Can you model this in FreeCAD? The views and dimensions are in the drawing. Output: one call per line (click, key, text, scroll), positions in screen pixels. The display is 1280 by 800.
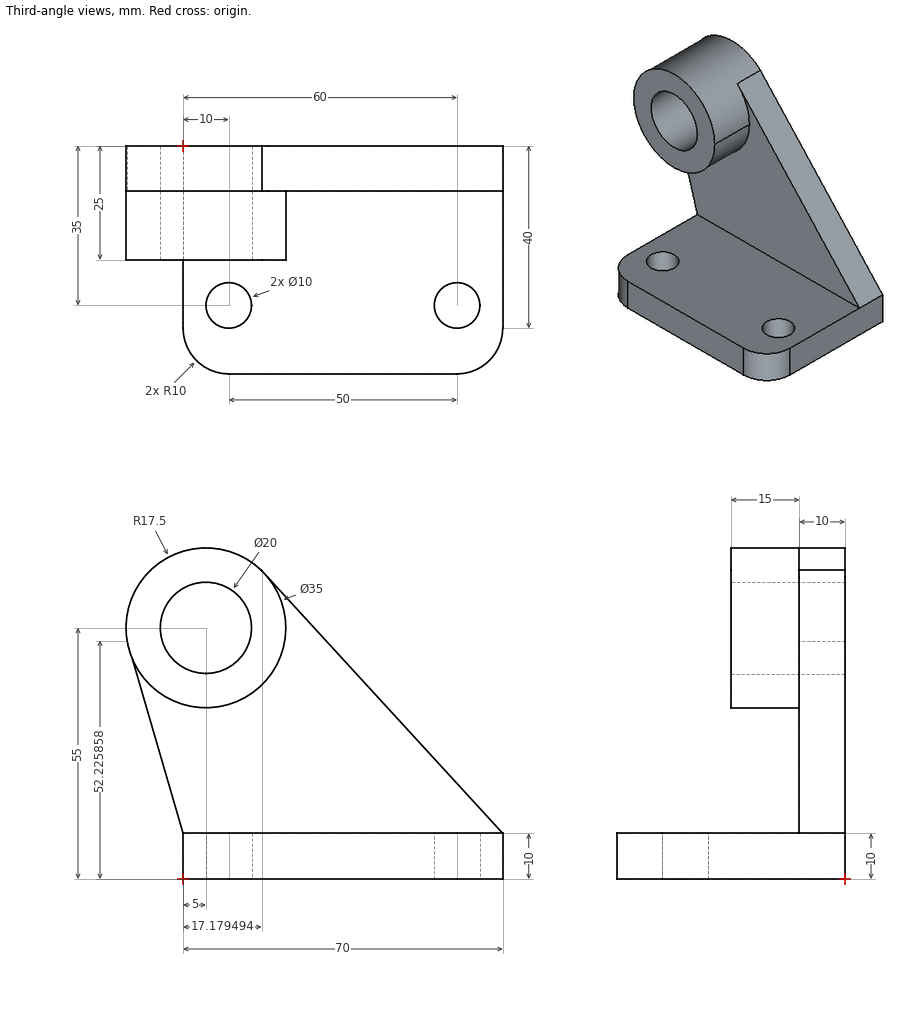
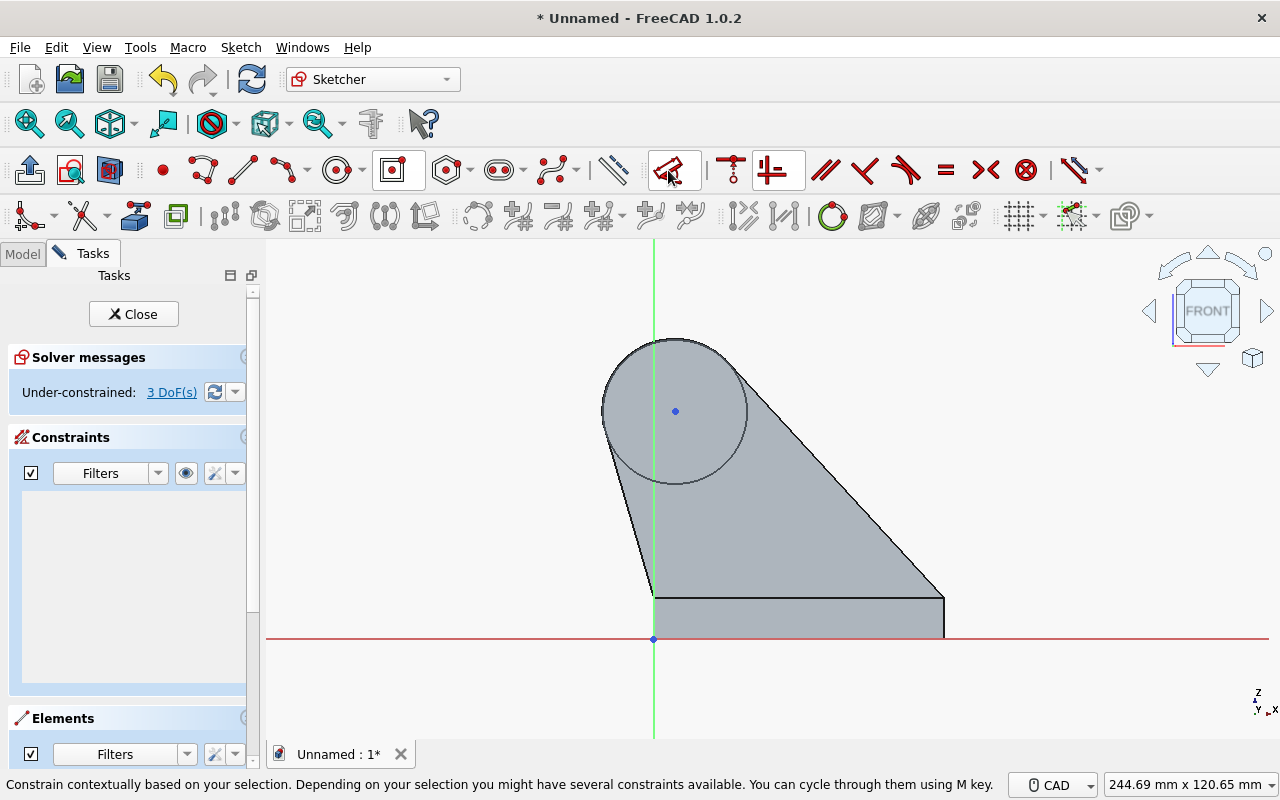
click(726, 361)
click(749, 338)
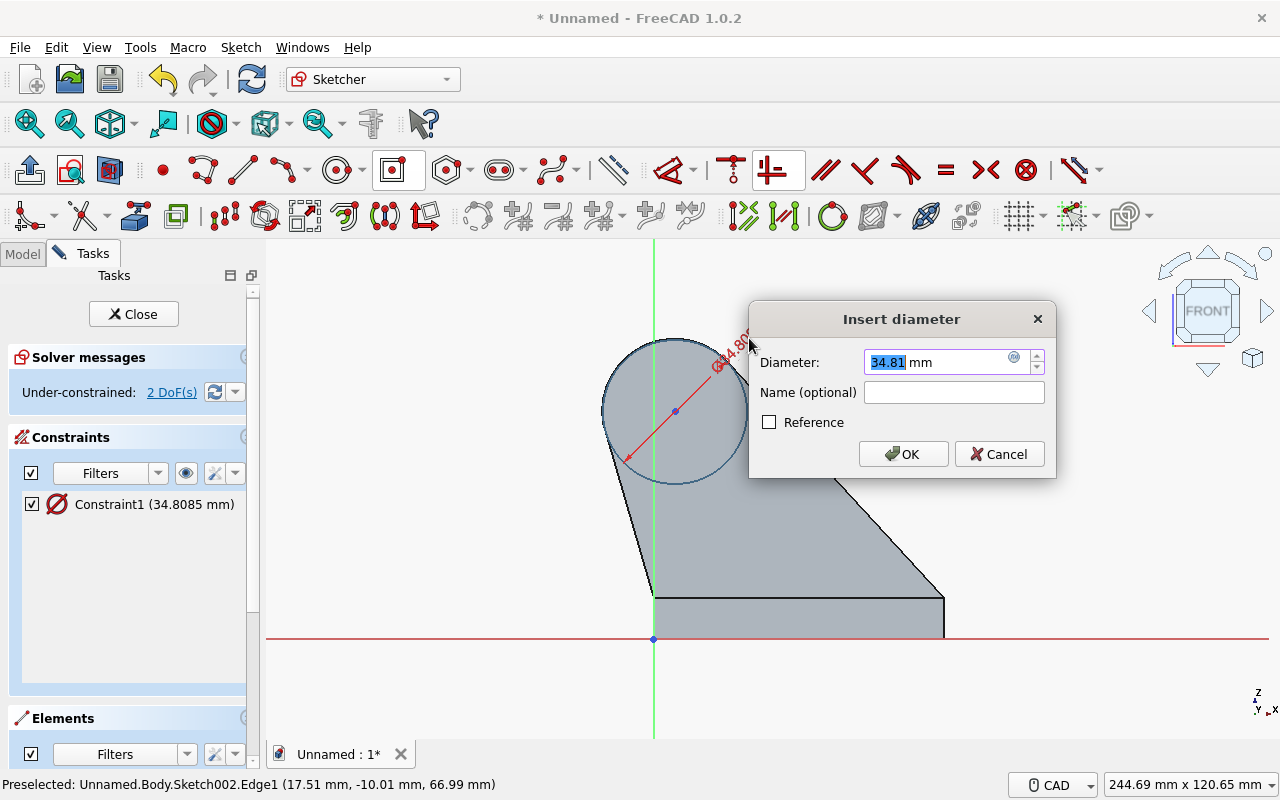
text(35)
key(Return)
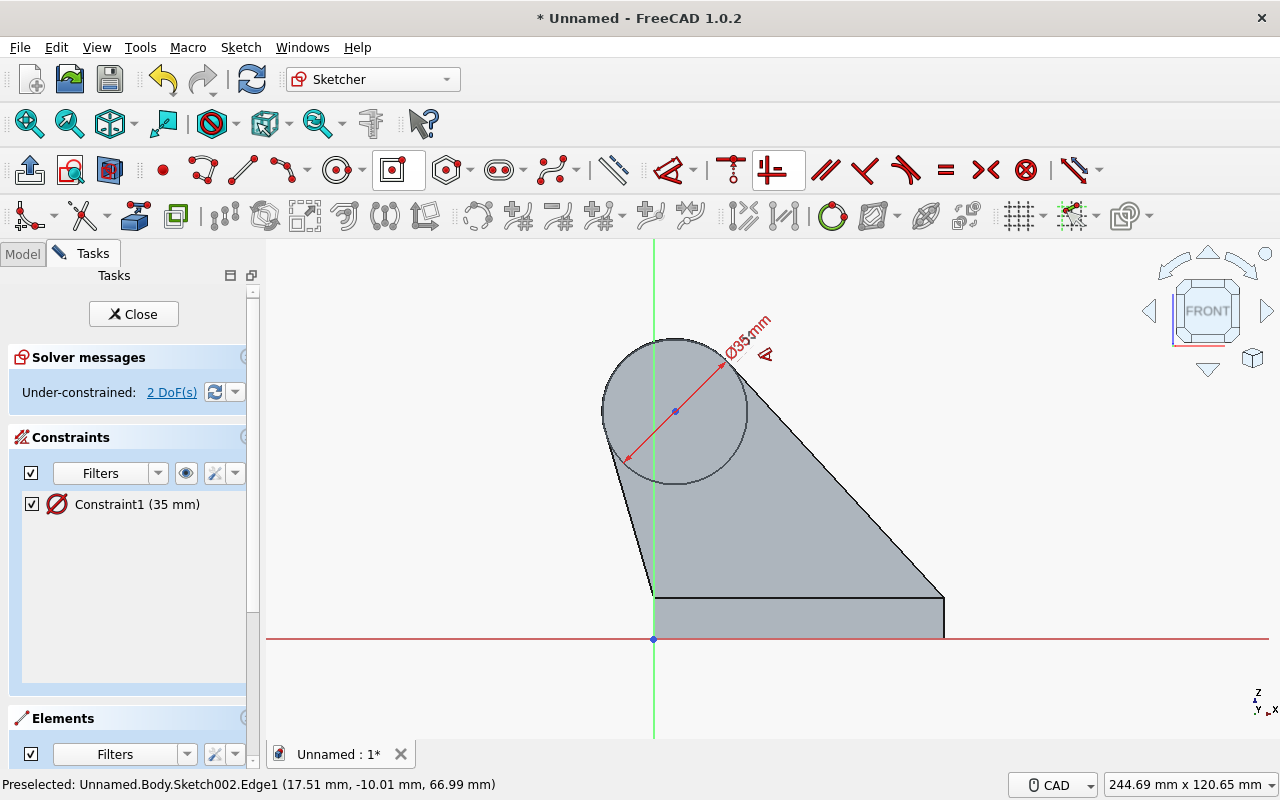
scroll(675, 412, up, 4)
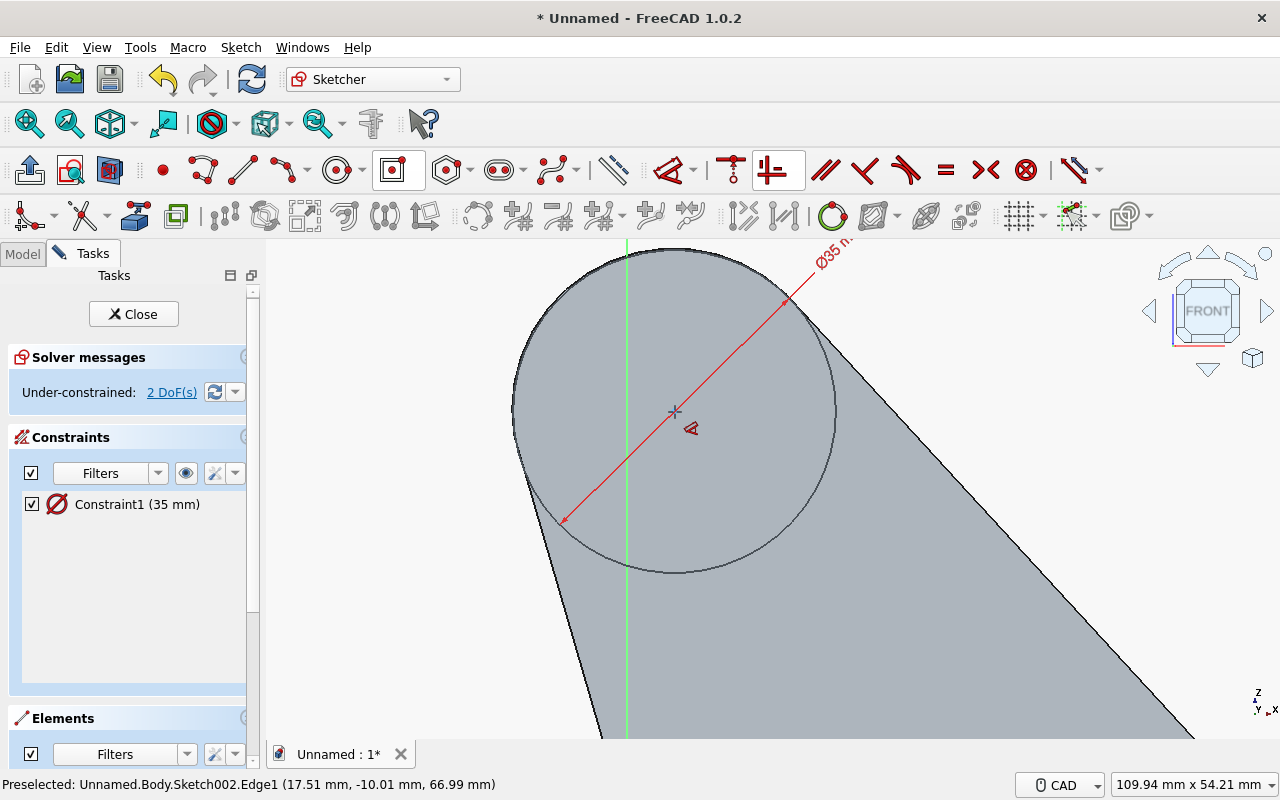
click(675, 412)
click(651, 378)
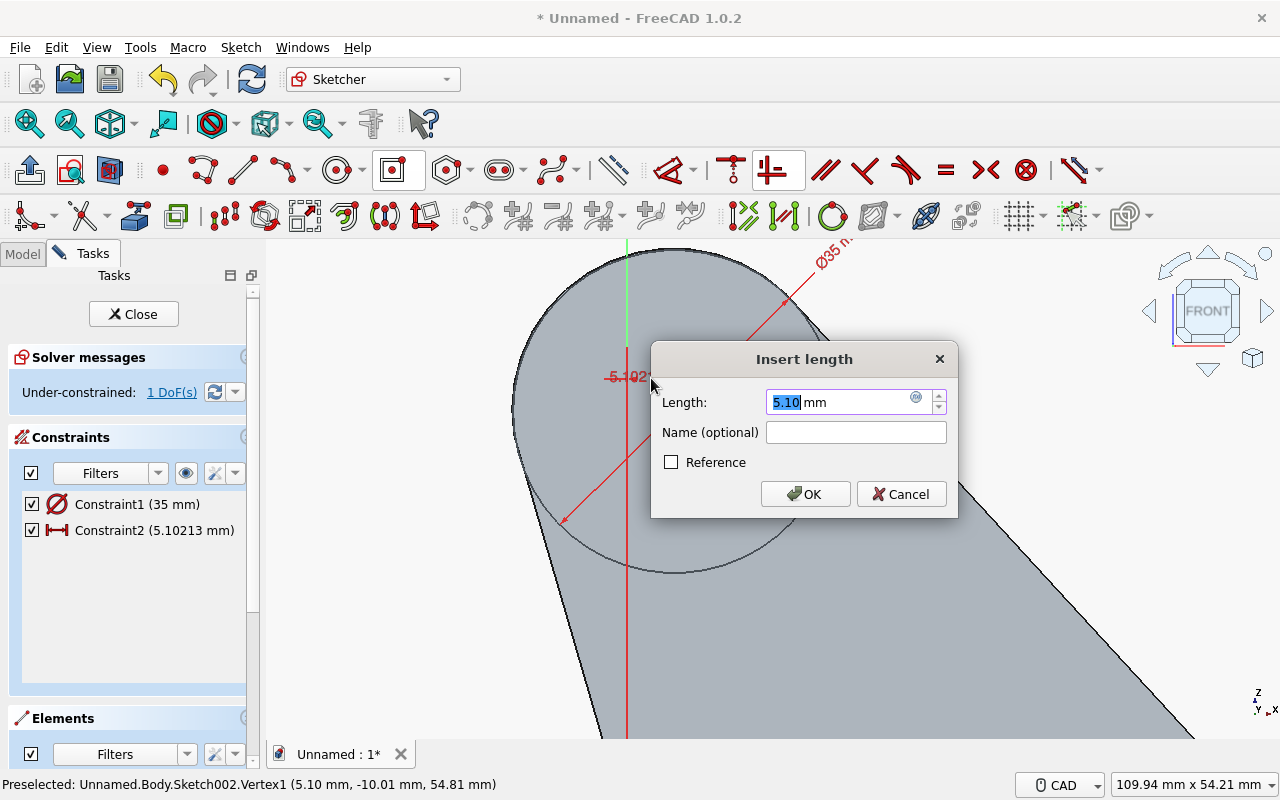
text(5)
key(Return)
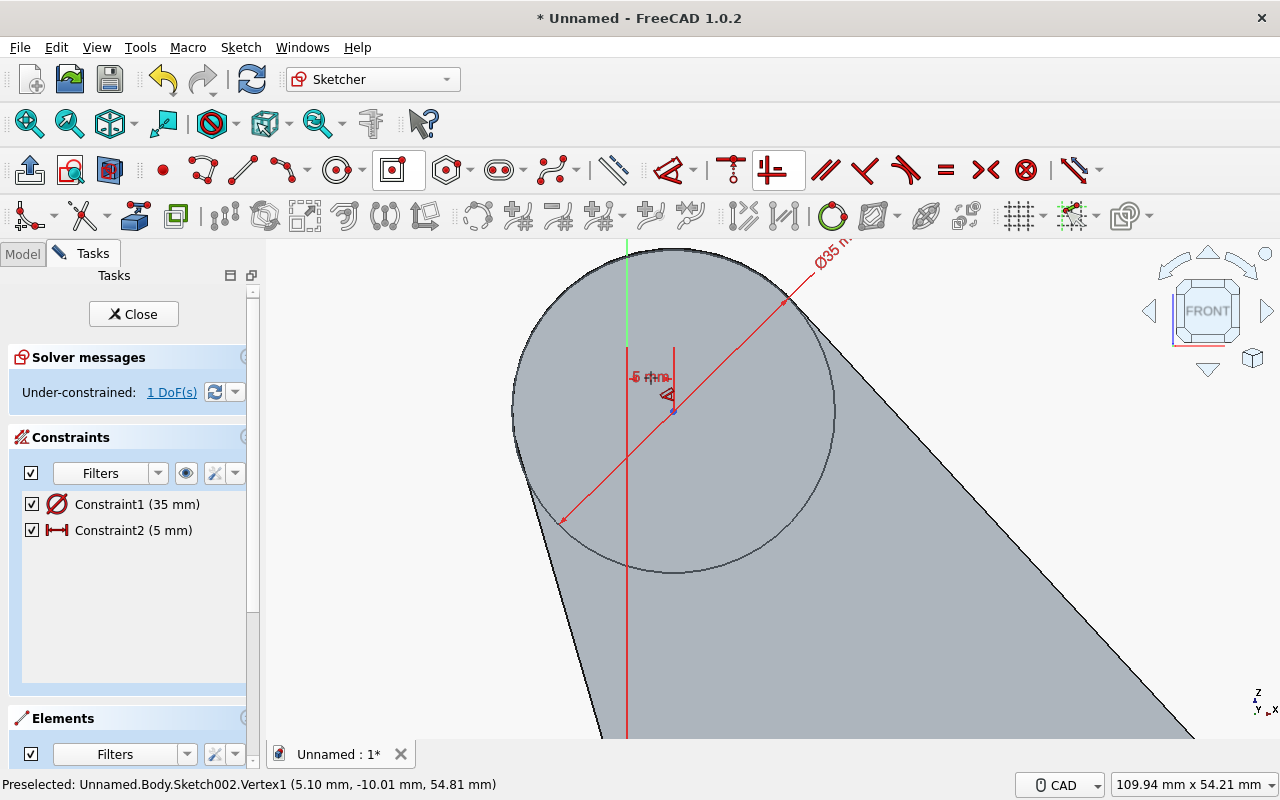
click(674, 412)
click(593, 492)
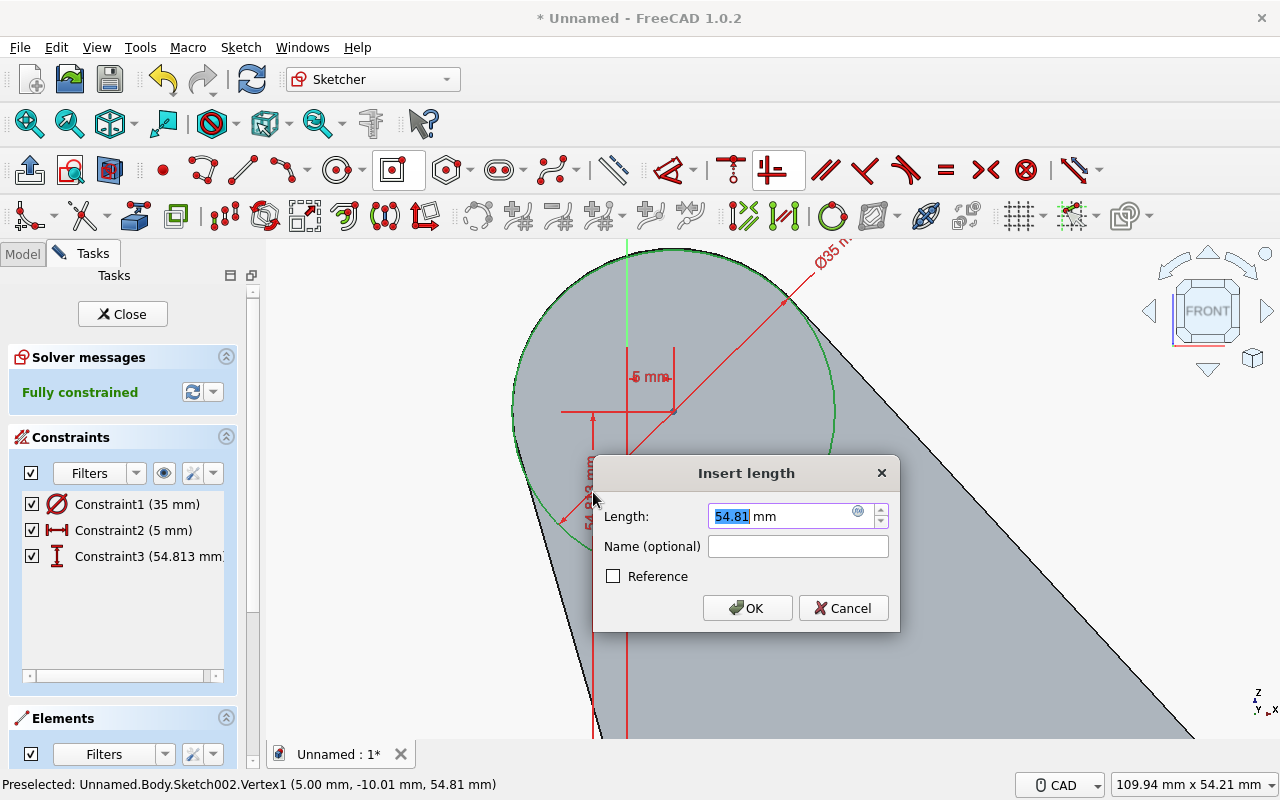
text(55)
key(Return)
key(Escape)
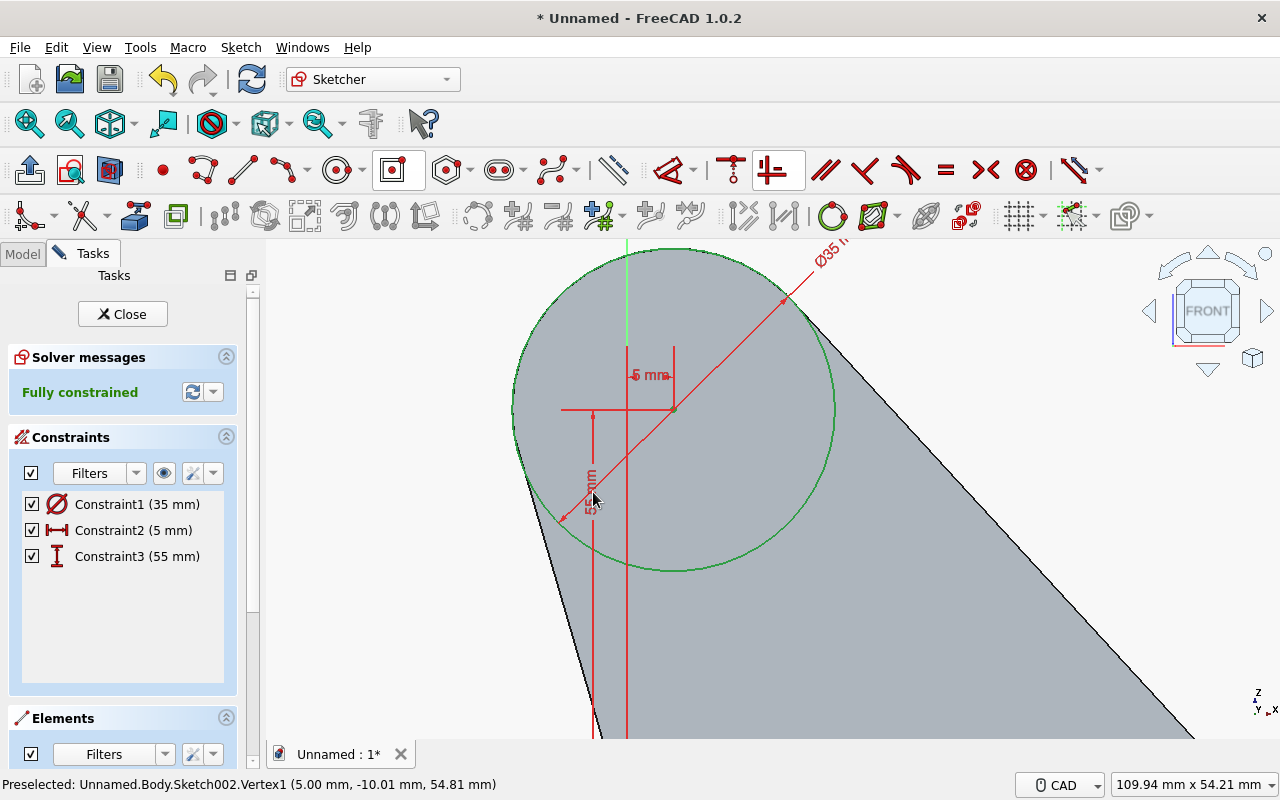
click(123, 314)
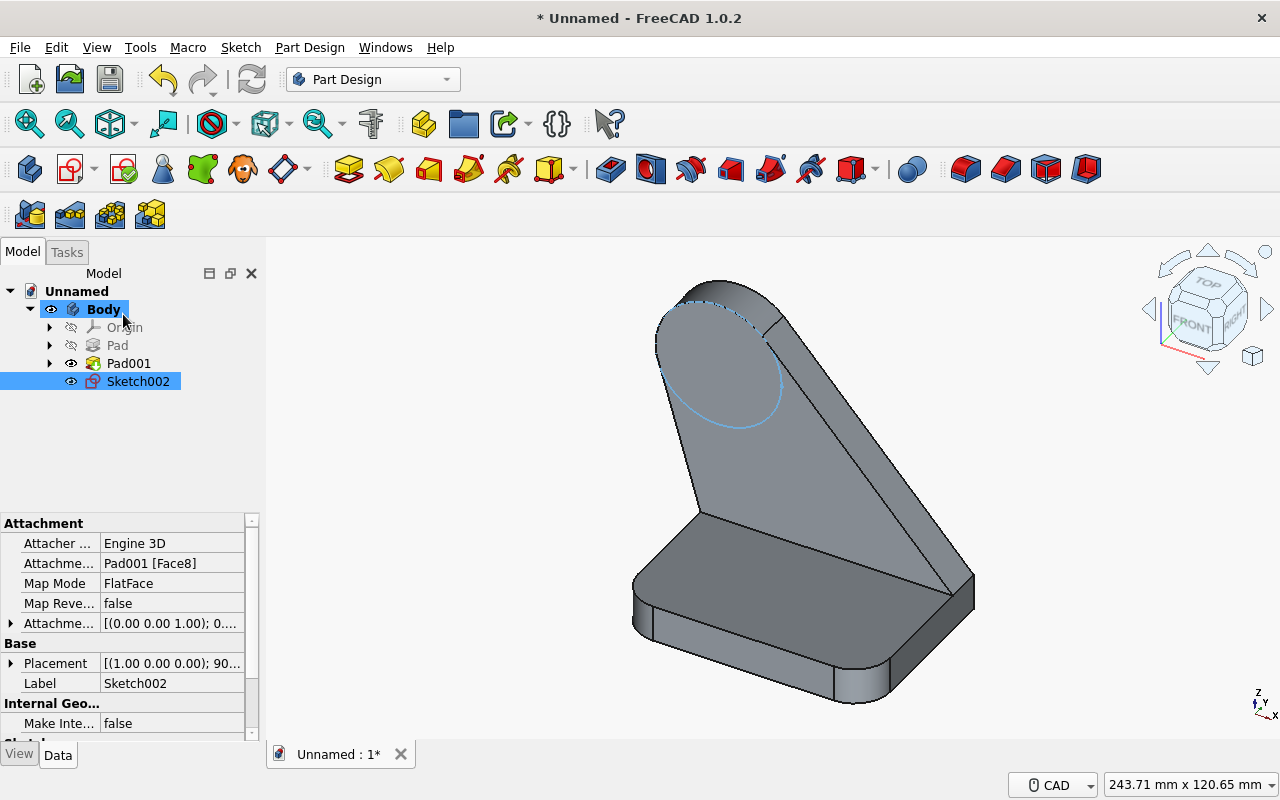
click(350, 170)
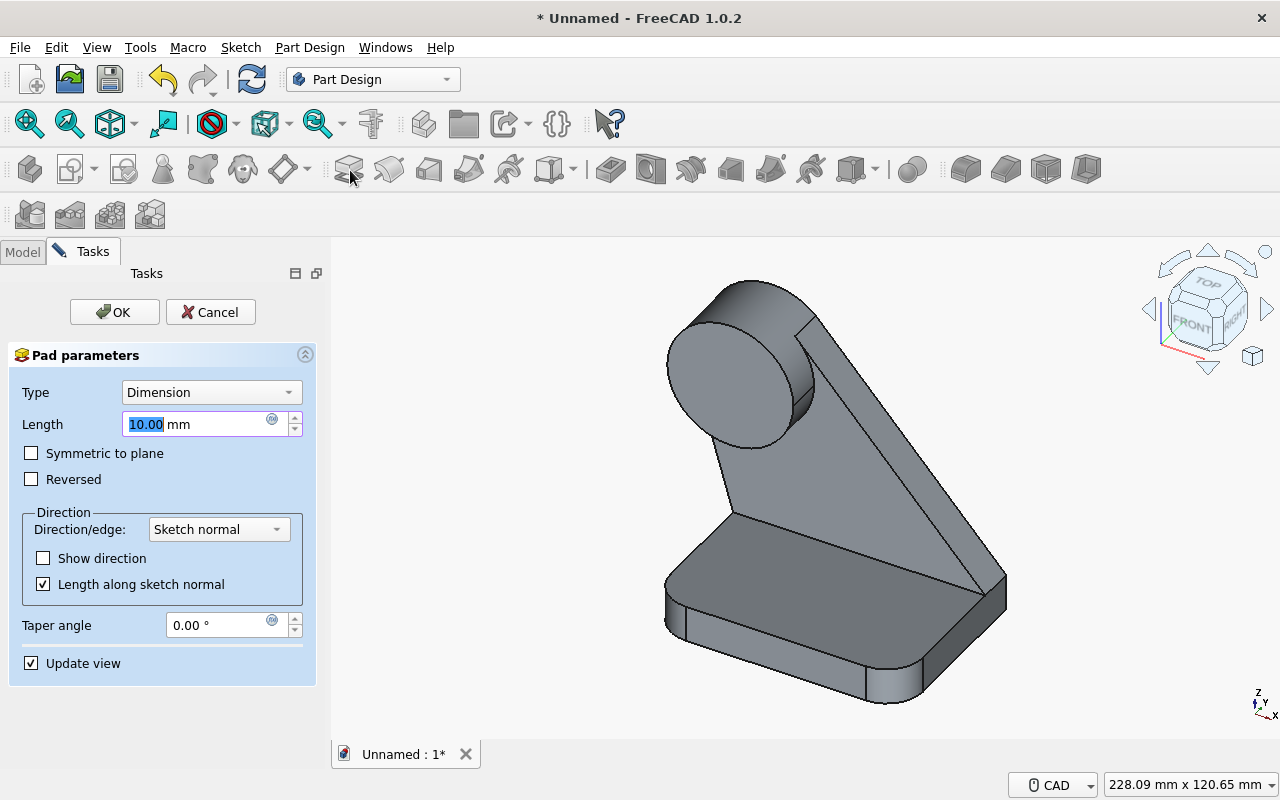
text(15)
key(Tab)